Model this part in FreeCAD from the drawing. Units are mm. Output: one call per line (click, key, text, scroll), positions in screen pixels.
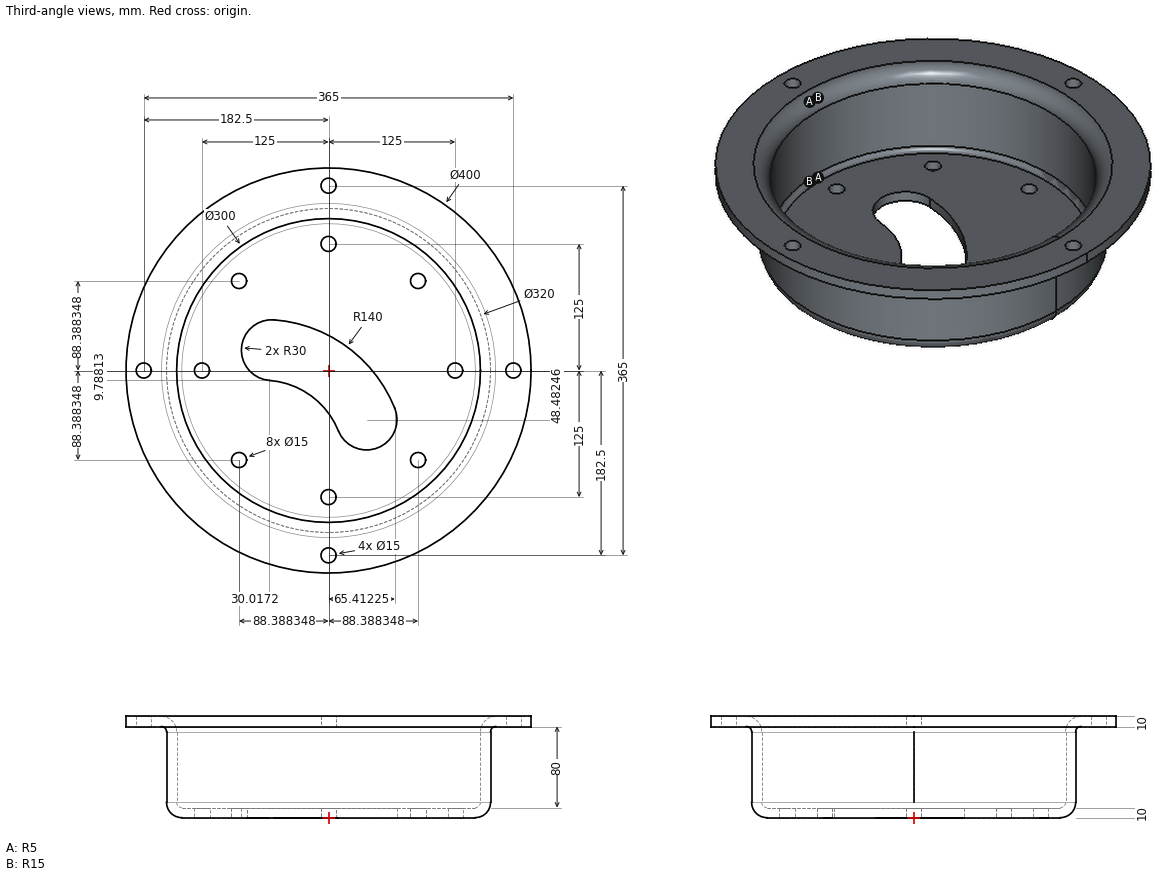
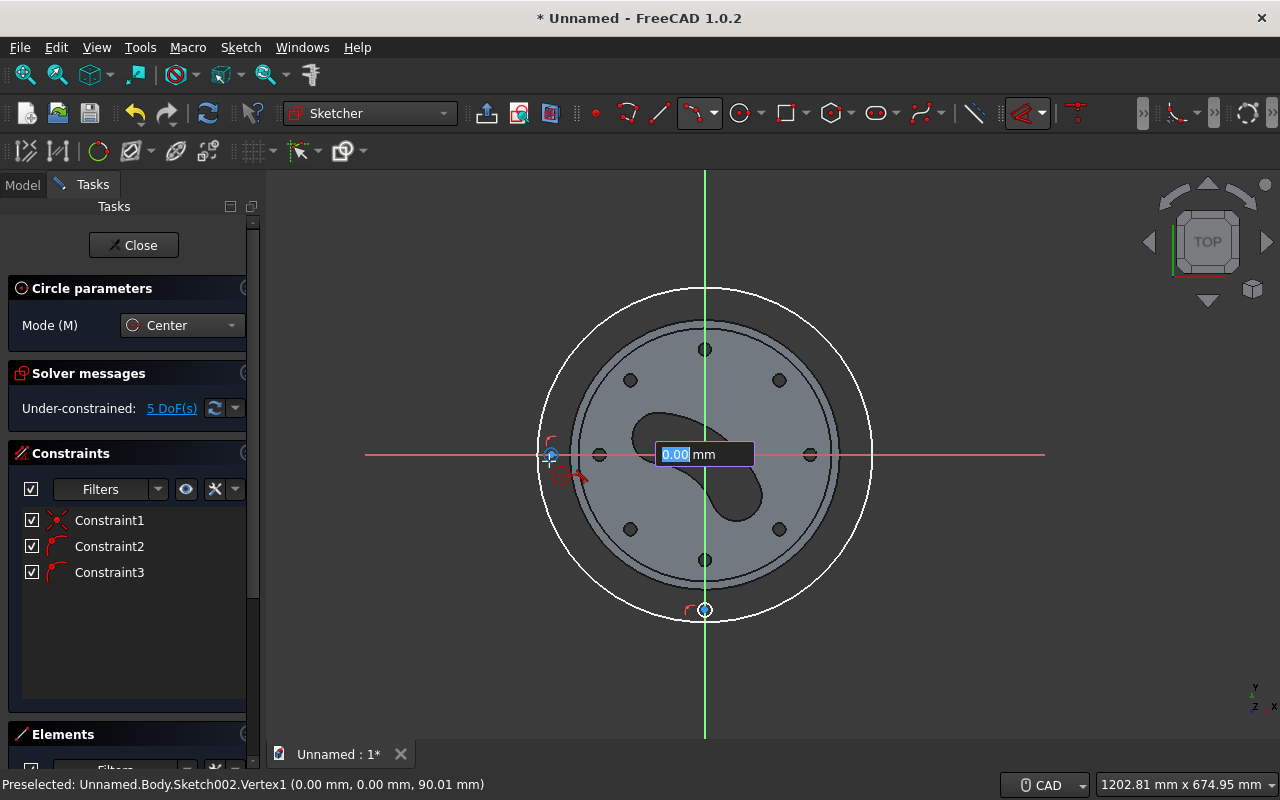
click(794, 365)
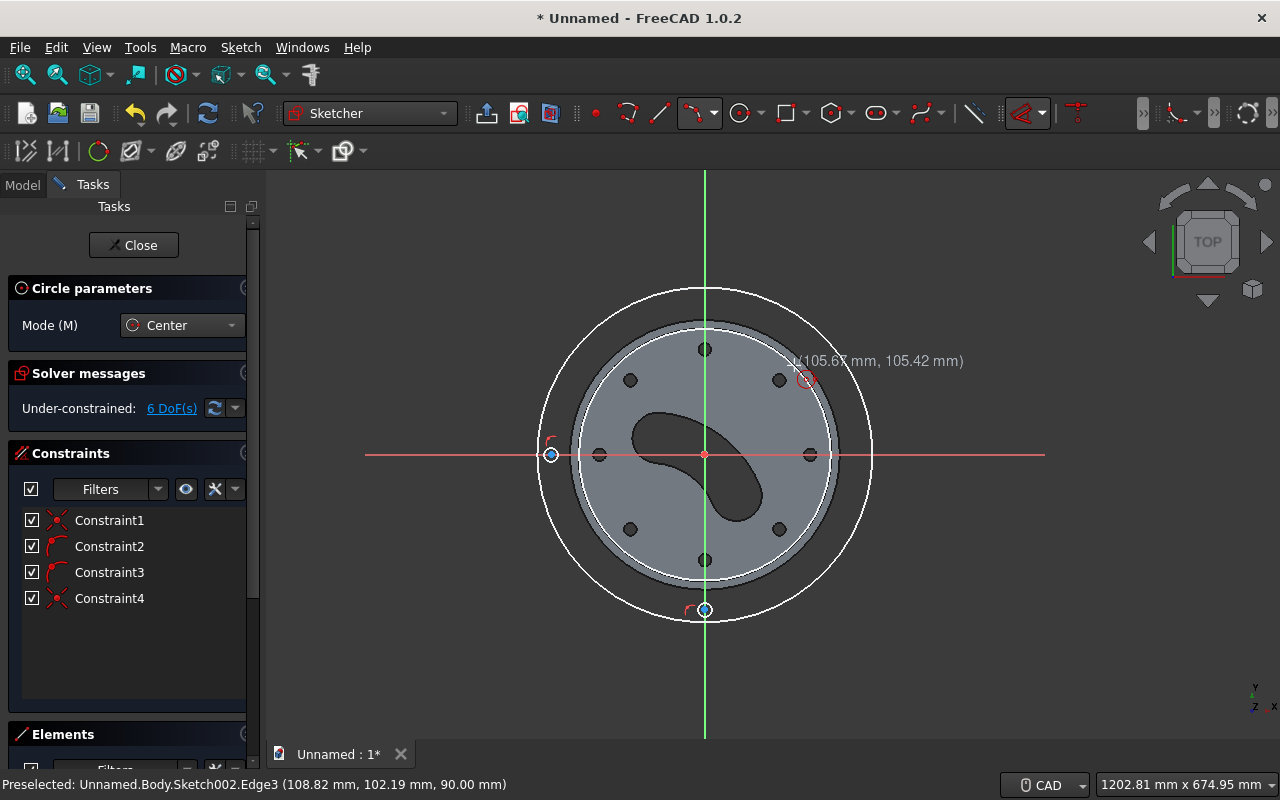
scroll(859, 455, up, 7)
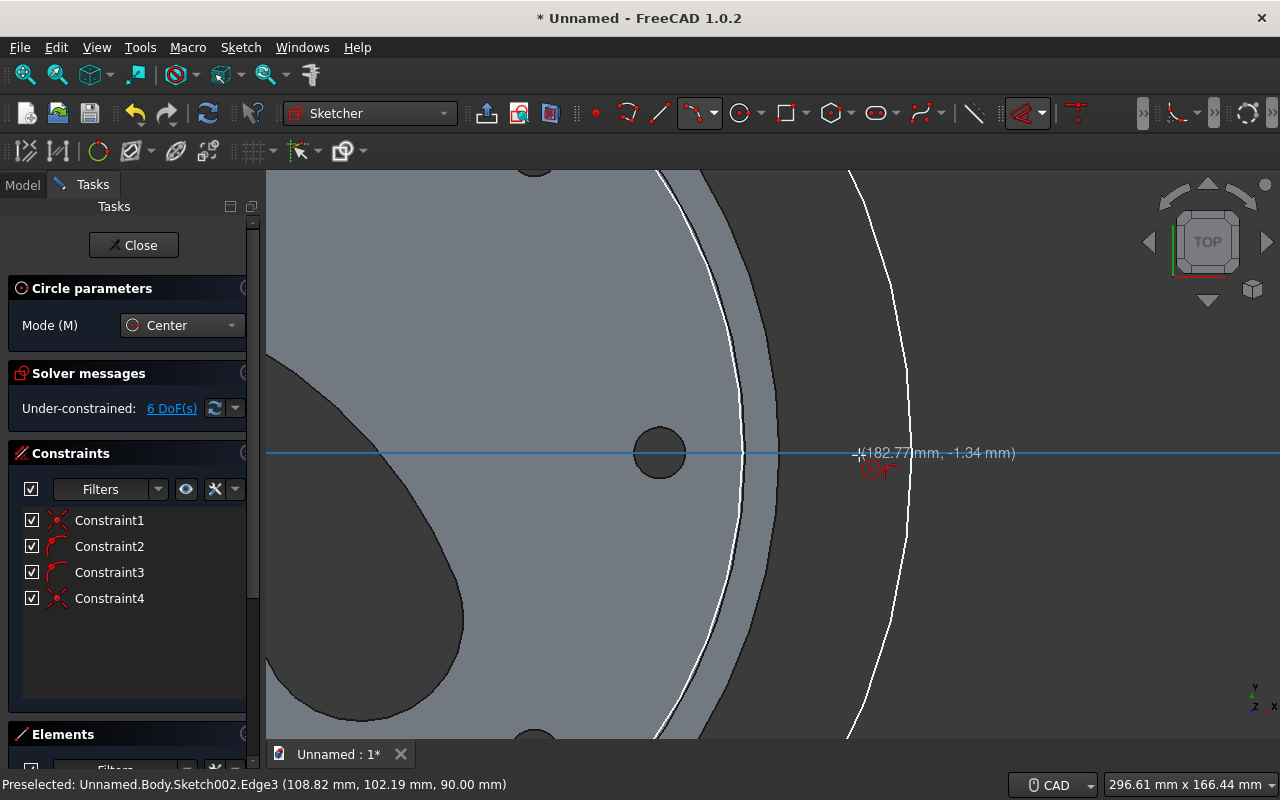
scroll(859, 455, down, 7)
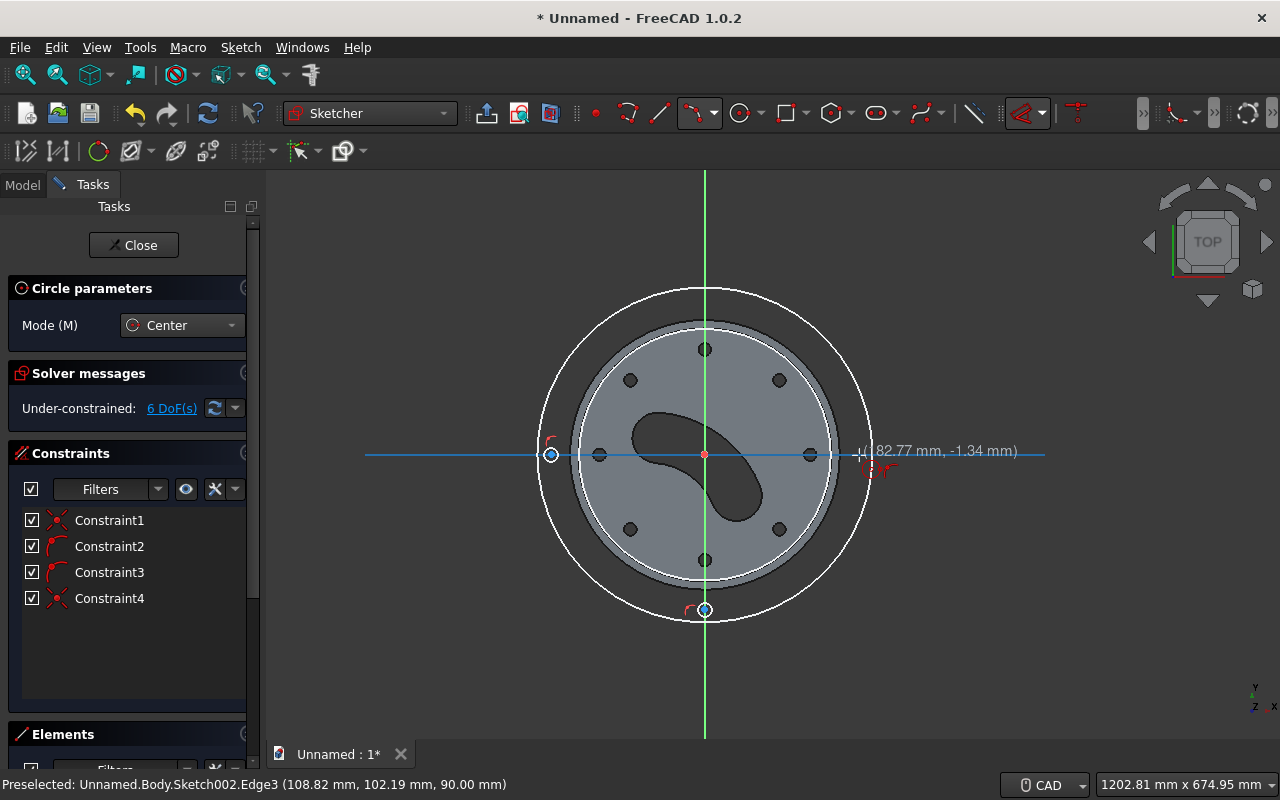
click(859, 455)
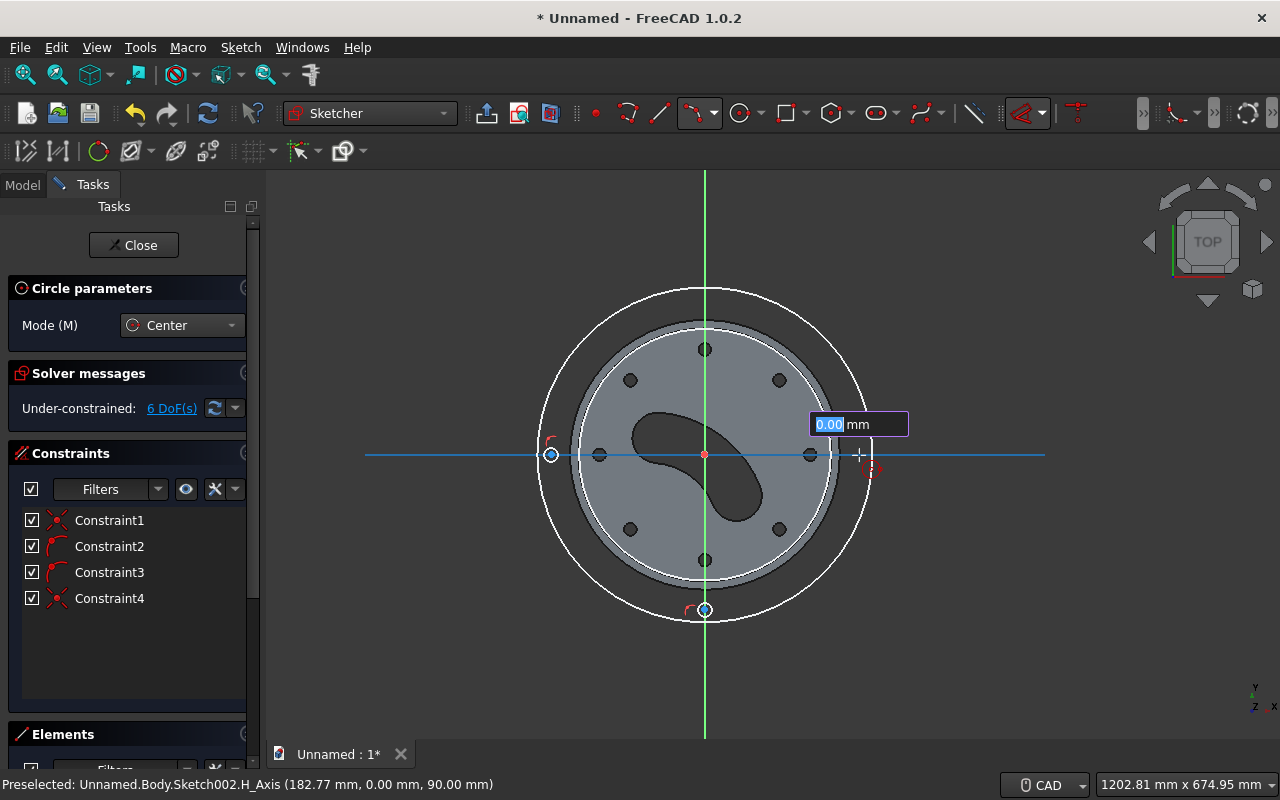
scroll(857, 461, up, 5)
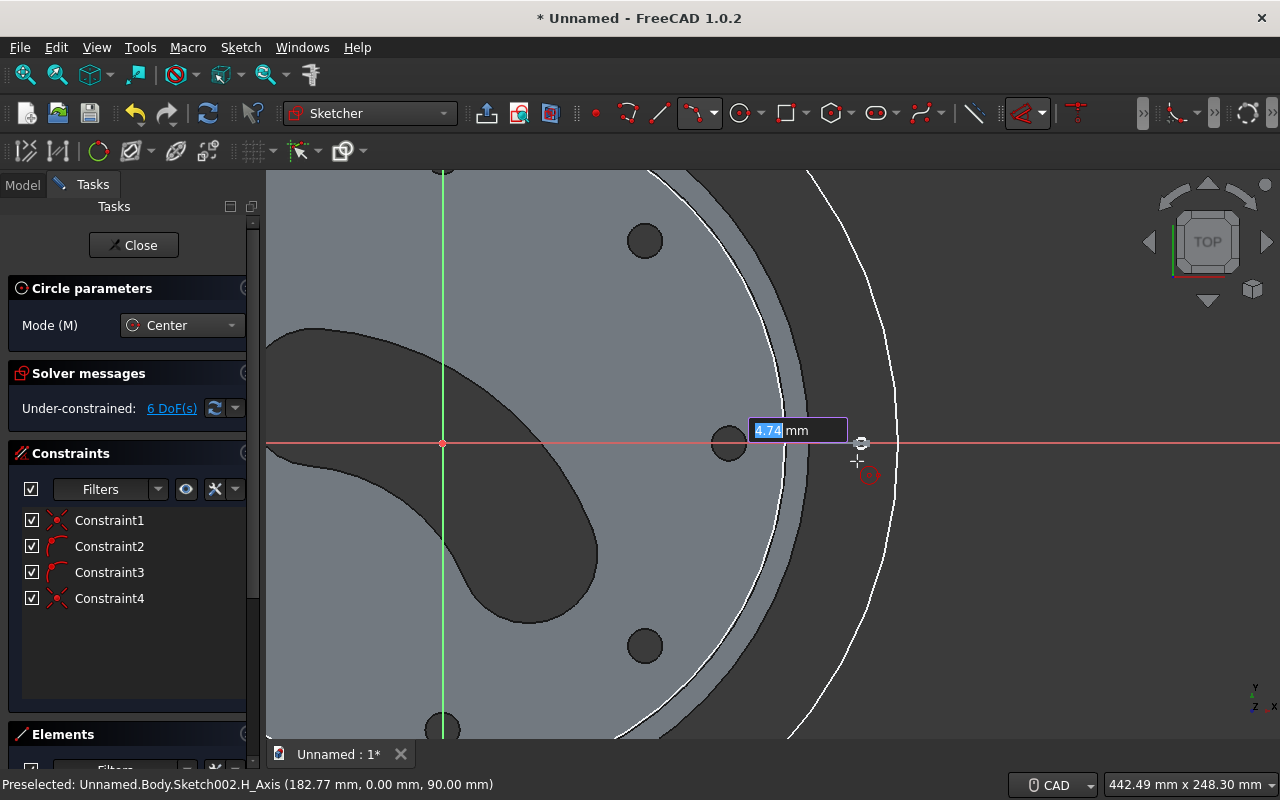
click(855, 460)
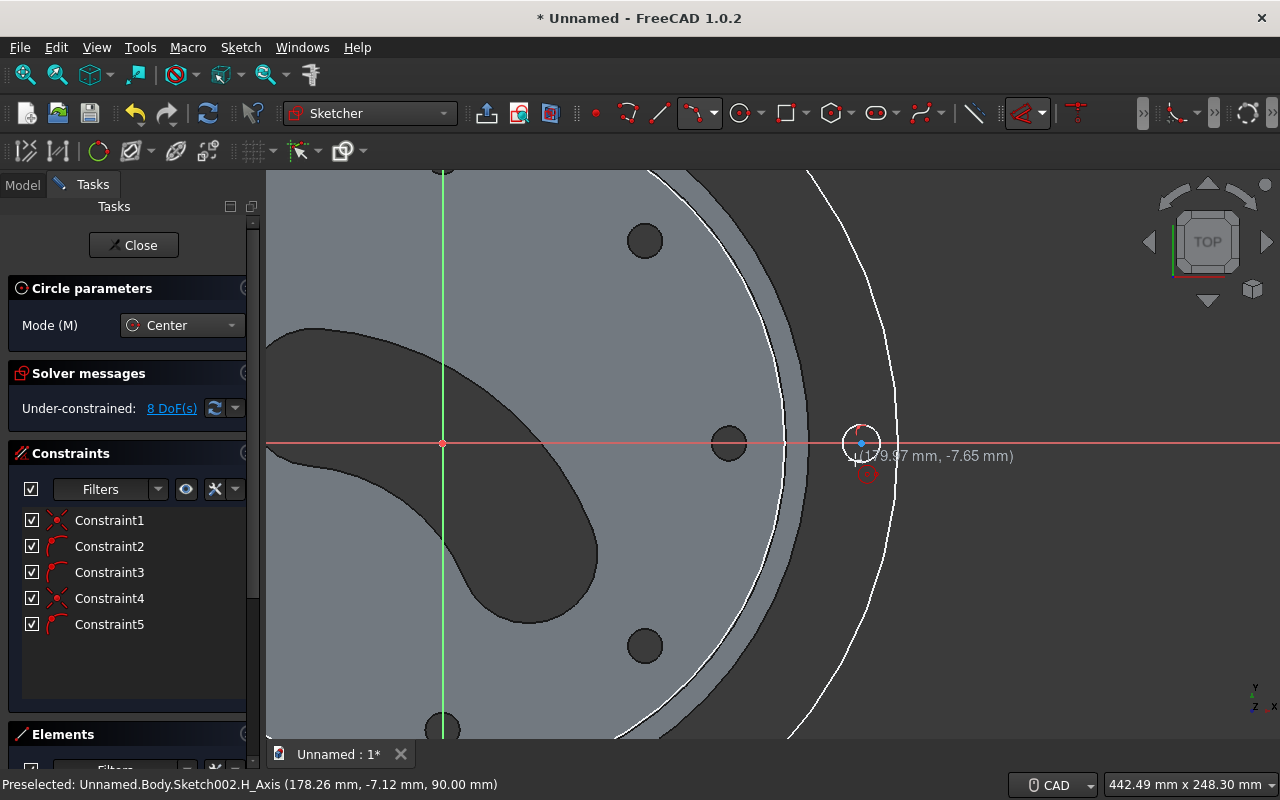
scroll(857, 461, down, 5)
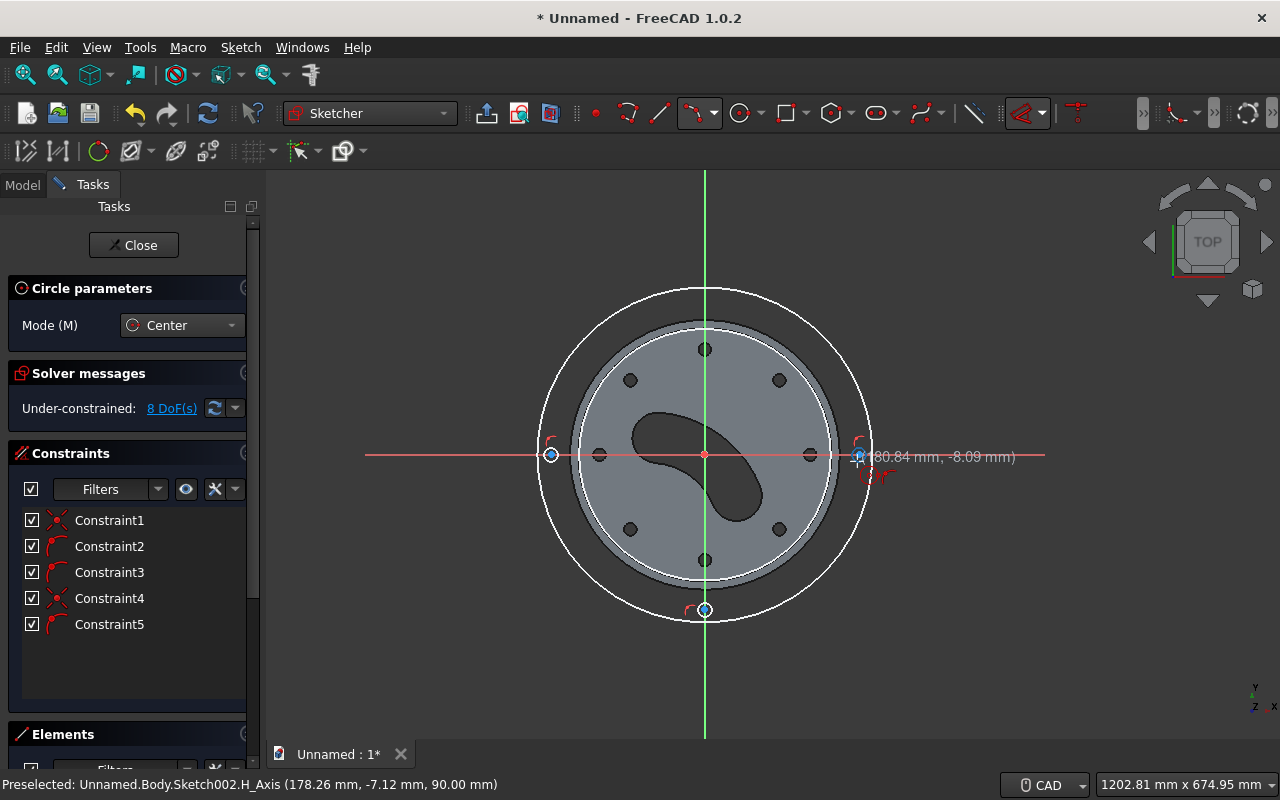
scroll(705, 301, up, 7)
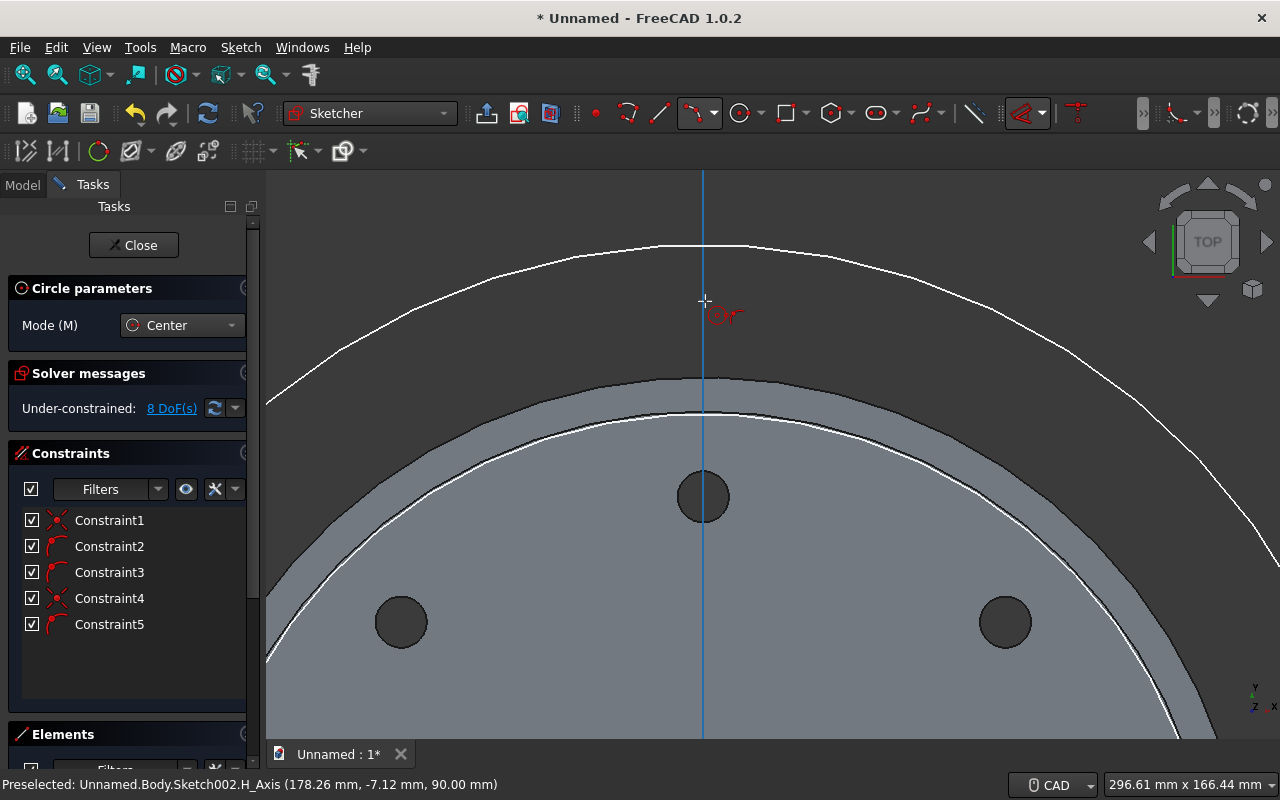
scroll(705, 301, down, 7)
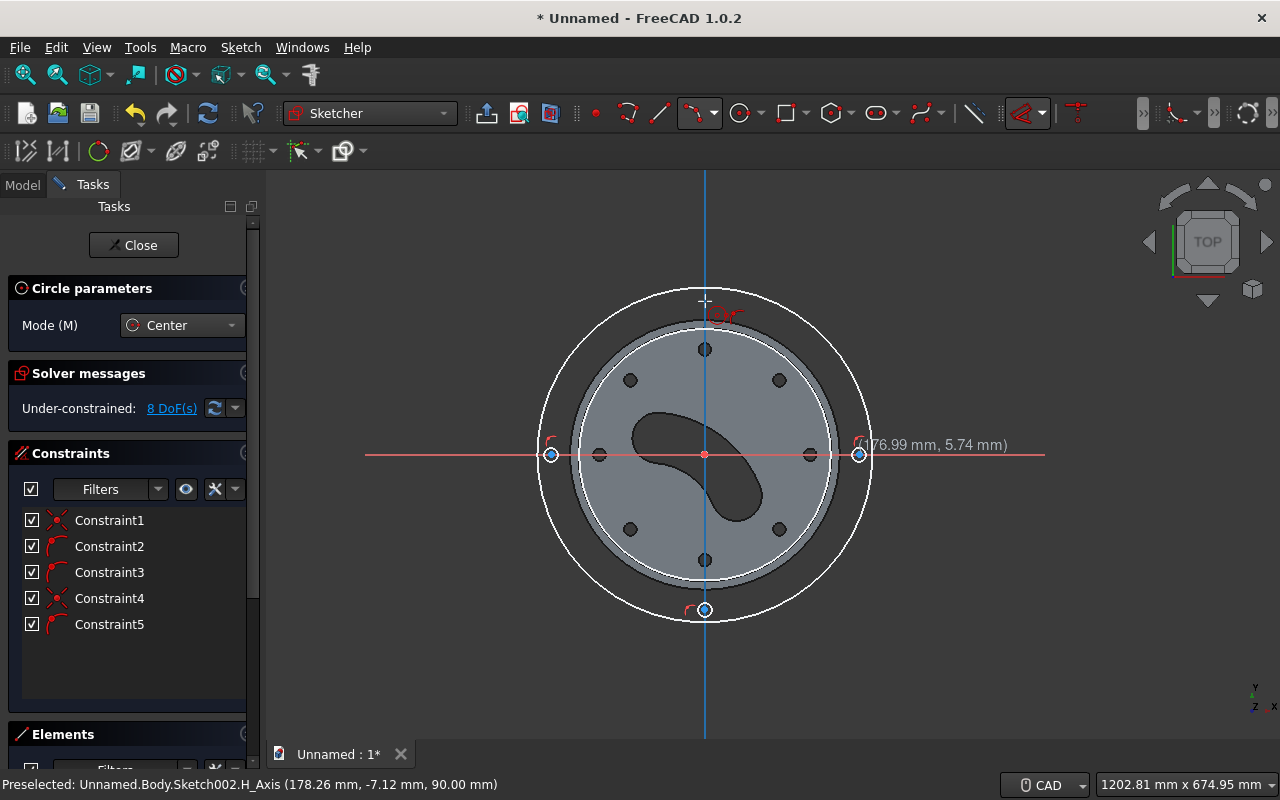
click(705, 301)